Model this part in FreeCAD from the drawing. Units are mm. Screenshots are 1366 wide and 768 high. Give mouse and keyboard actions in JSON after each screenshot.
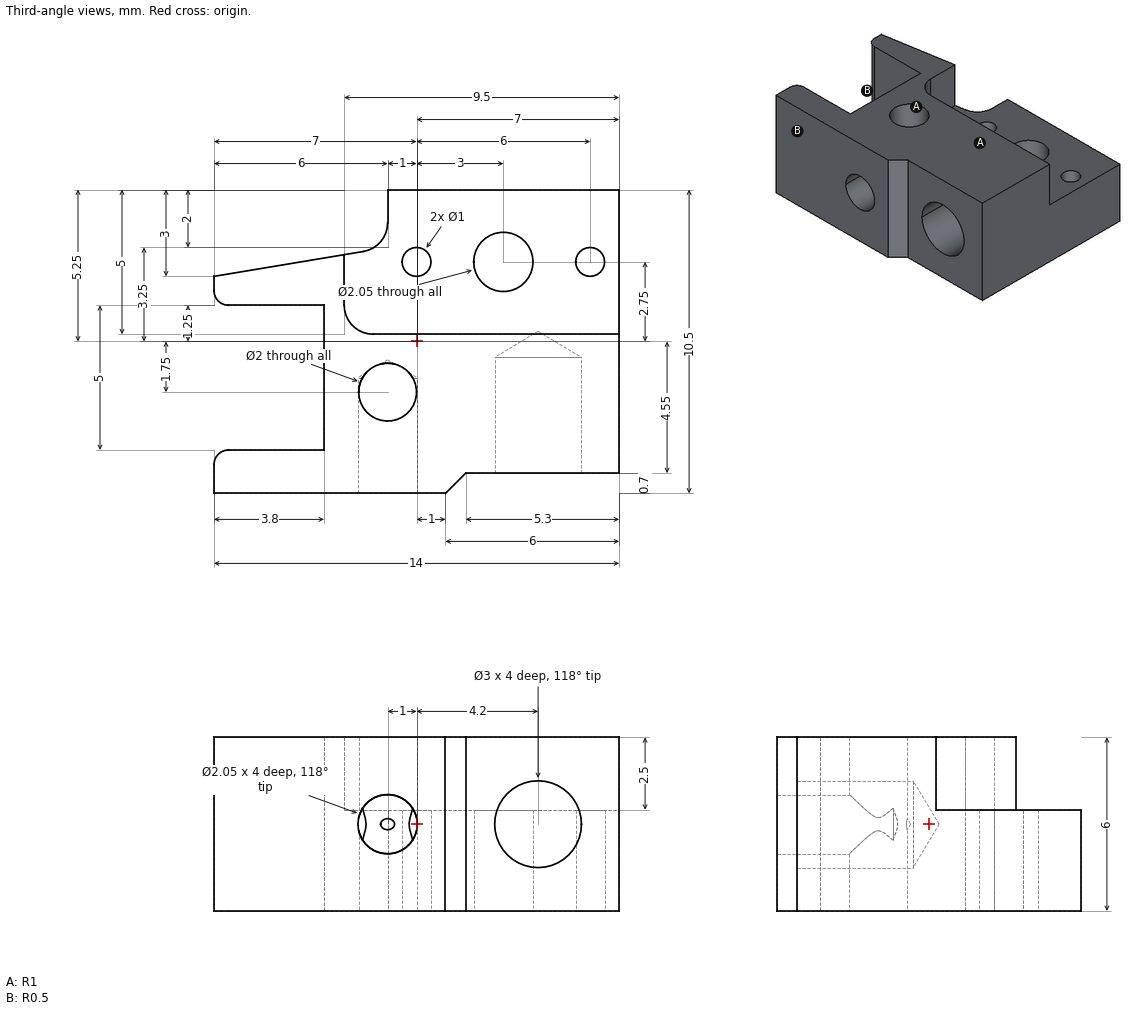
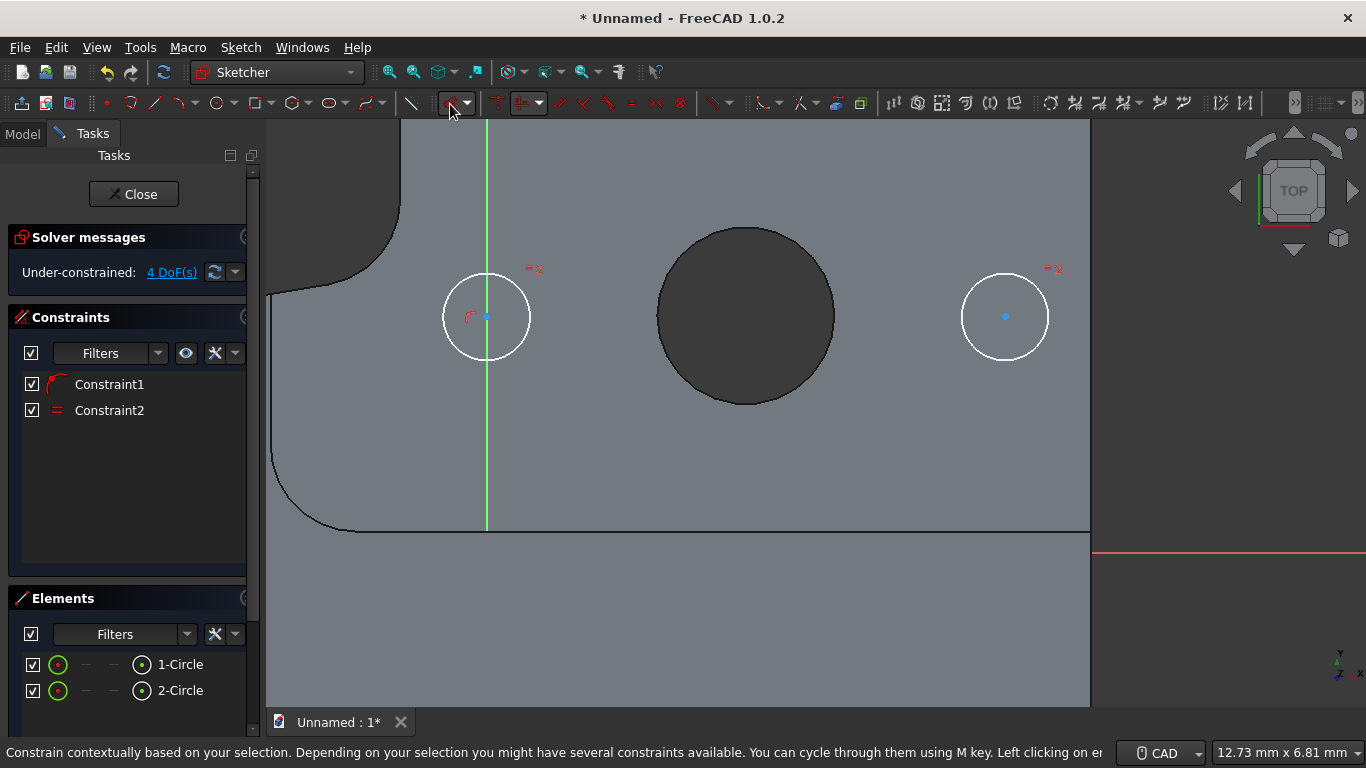
{"action": "left_click", "coordinate": [517, 286]}
{"action": "left_click", "coordinate": [539, 263]}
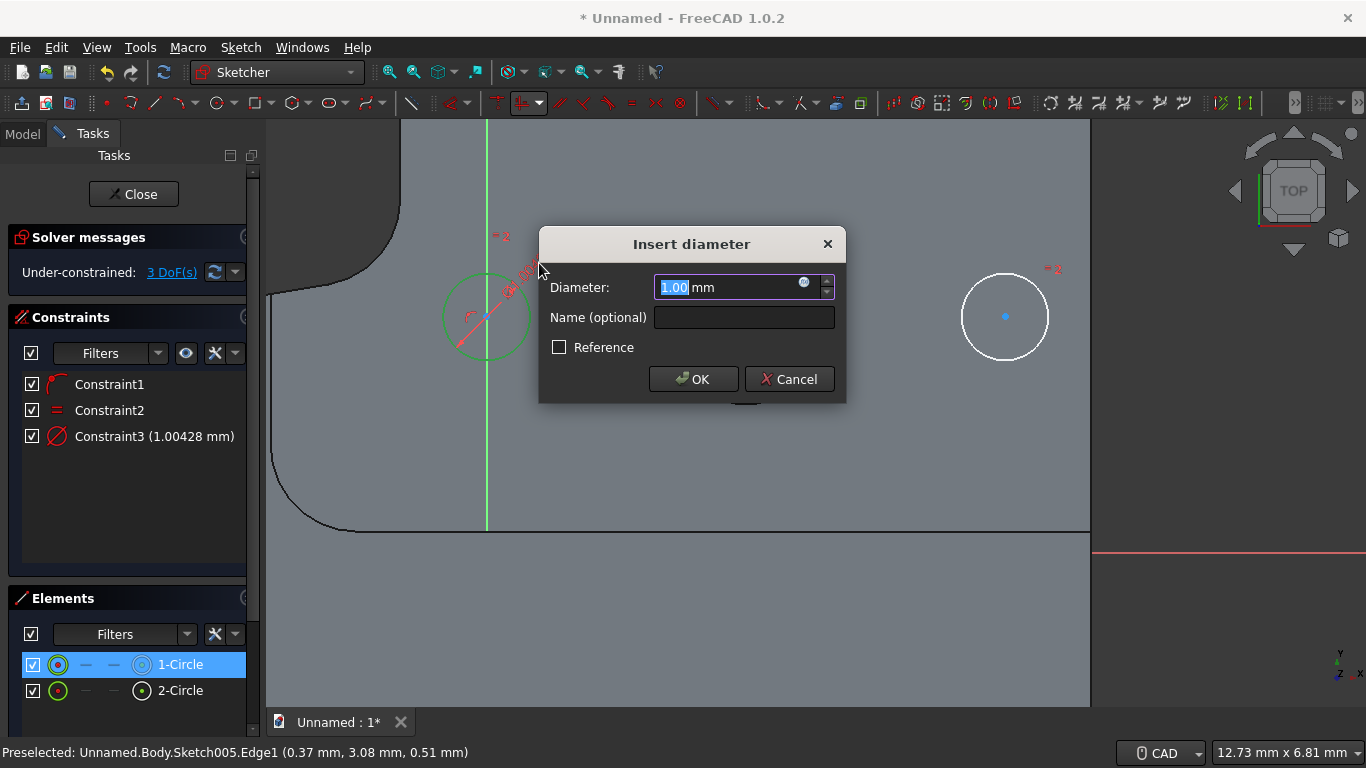
{"action": "type", "text": "1"}
{"action": "key", "text": "Return"}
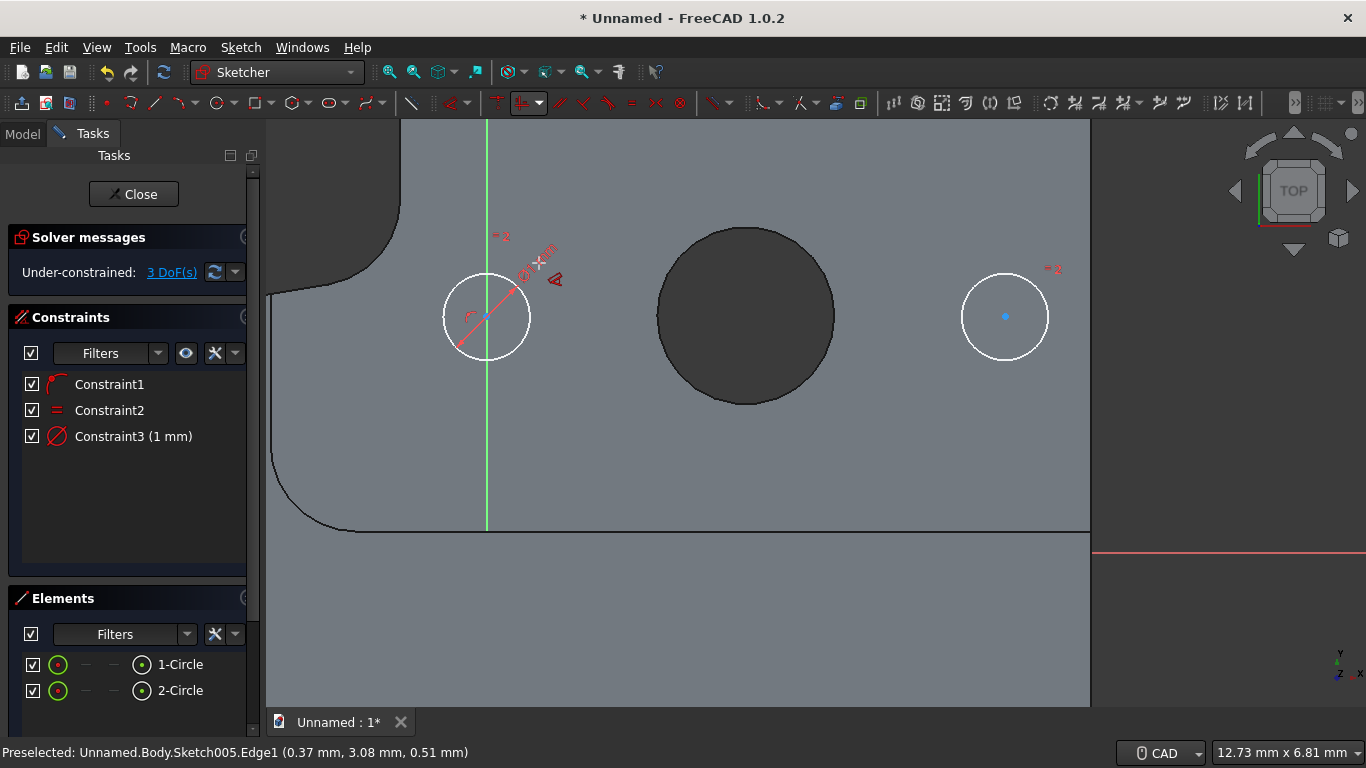
{"action": "left_click", "coordinate": [1005, 317]}
{"action": "left_click", "coordinate": [746, 587]}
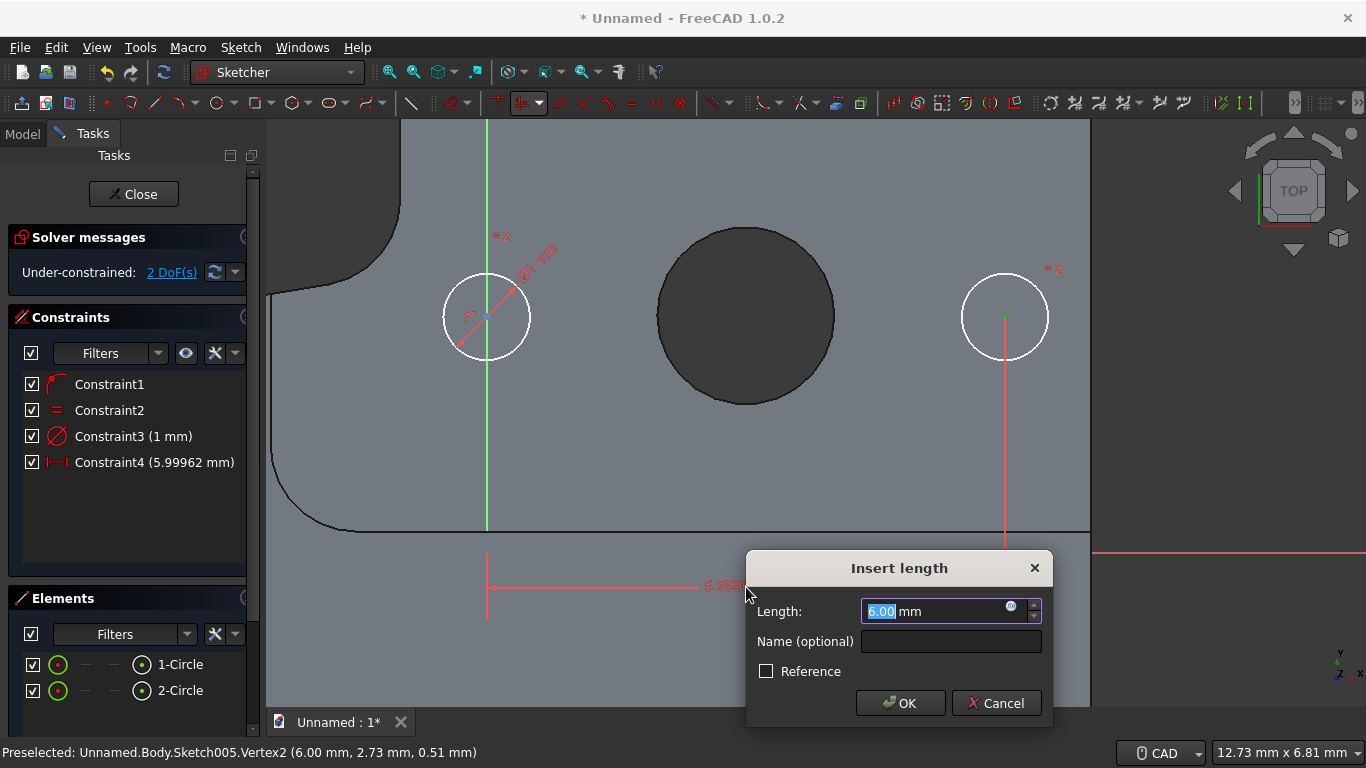
{"action": "type", "text": "6"}
{"action": "key", "text": "Return"}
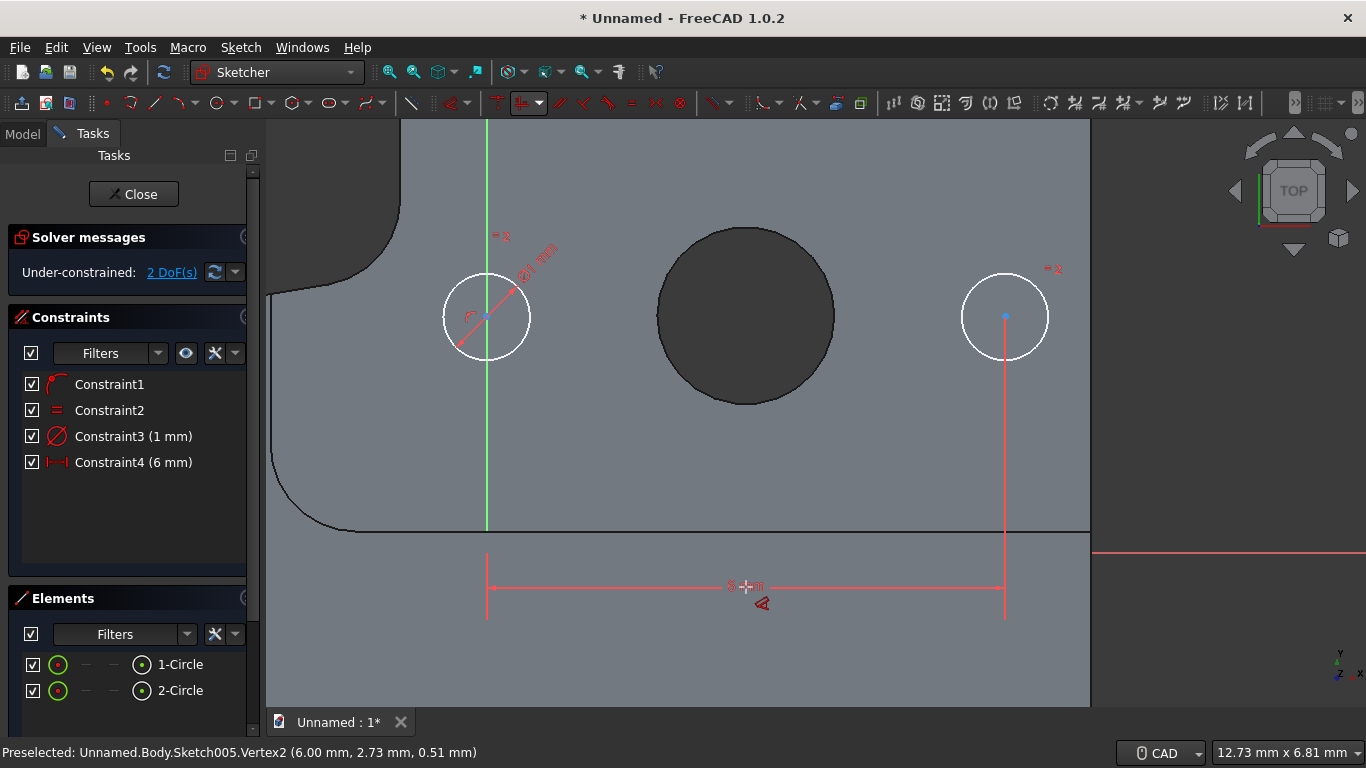
{"action": "left_click", "coordinate": [487, 317]}
{"action": "left_click", "coordinate": [453, 435]}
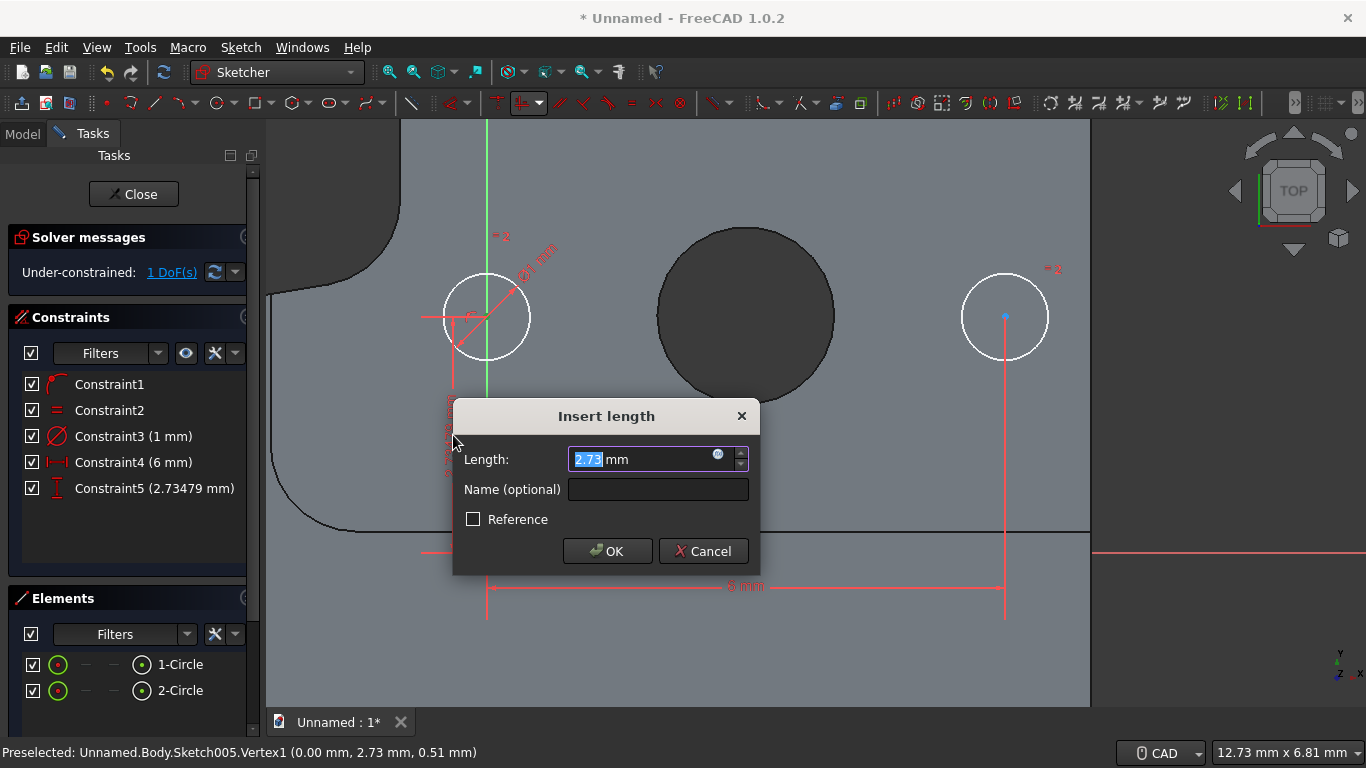
{"action": "type", "text": "2.75"}
{"action": "key", "text": "Return"}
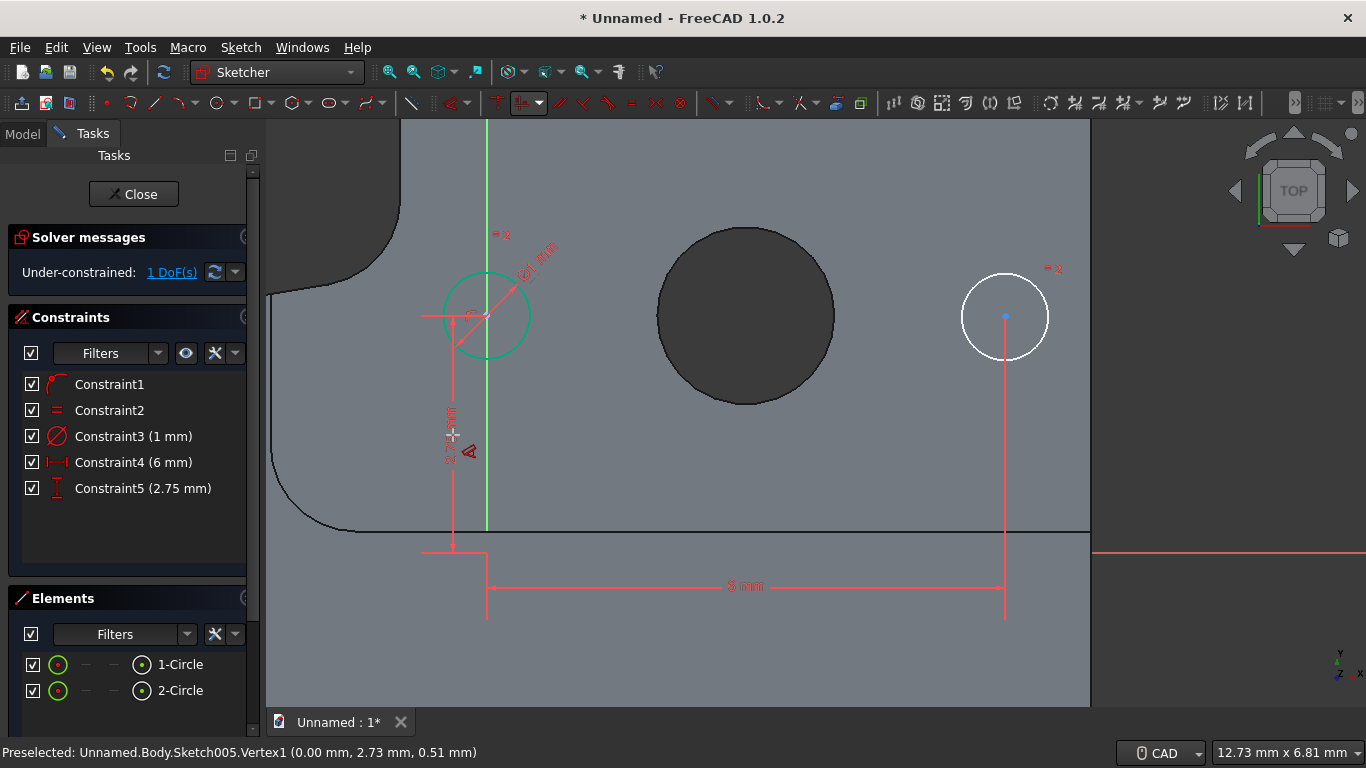
{"action": "left_click", "coordinate": [1005, 317]}
{"action": "left_click", "coordinate": [1039, 435]}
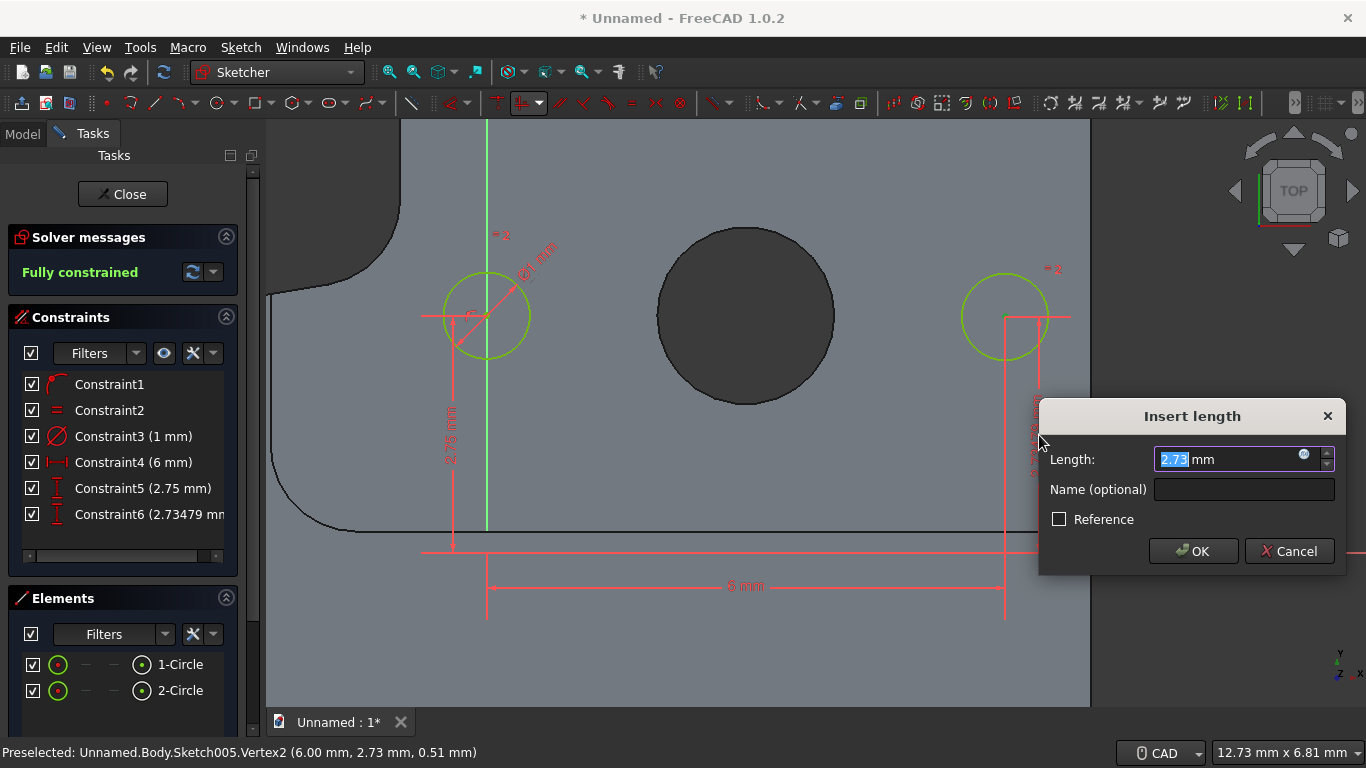
{"action": "type", "text": "2.75"}
{"action": "key", "text": "Return"}
{"action": "key", "text": "Escape"}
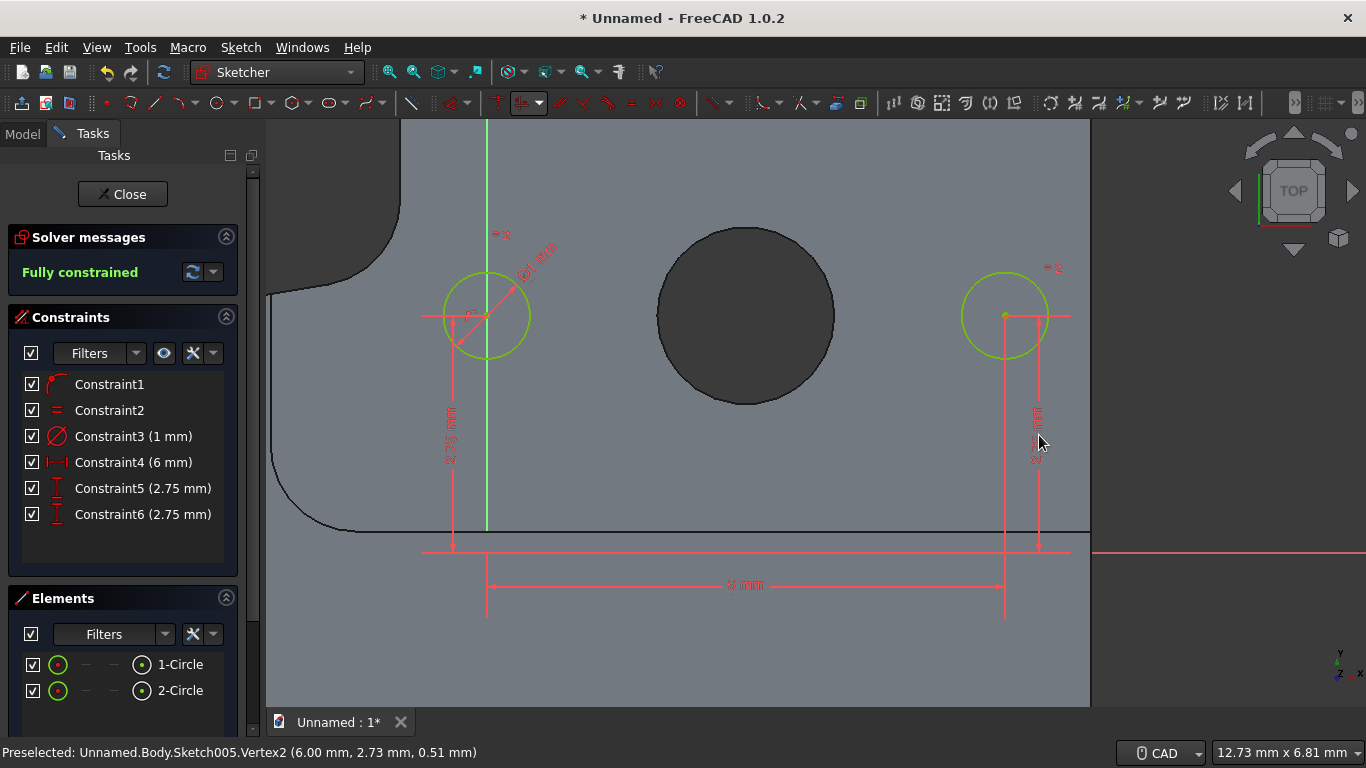
{"action": "left_click", "coordinate": [123, 194]}